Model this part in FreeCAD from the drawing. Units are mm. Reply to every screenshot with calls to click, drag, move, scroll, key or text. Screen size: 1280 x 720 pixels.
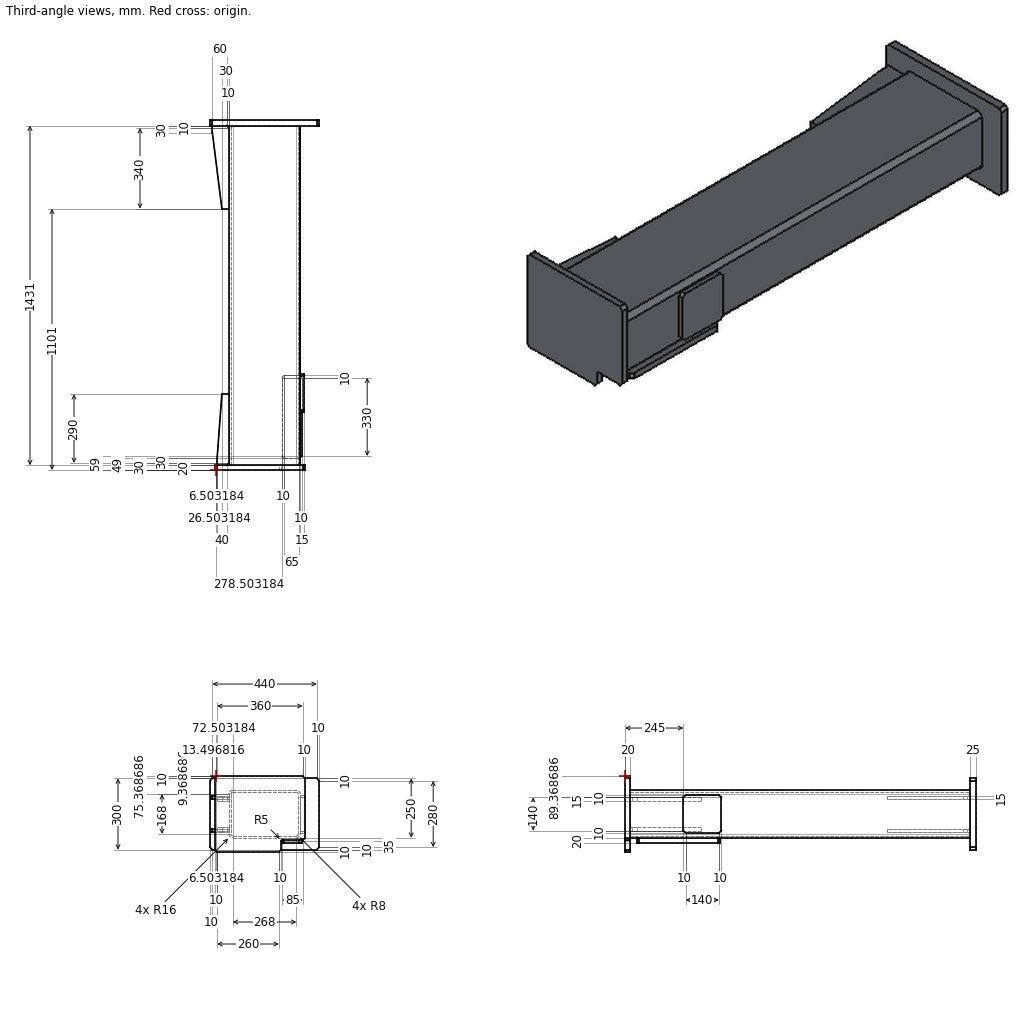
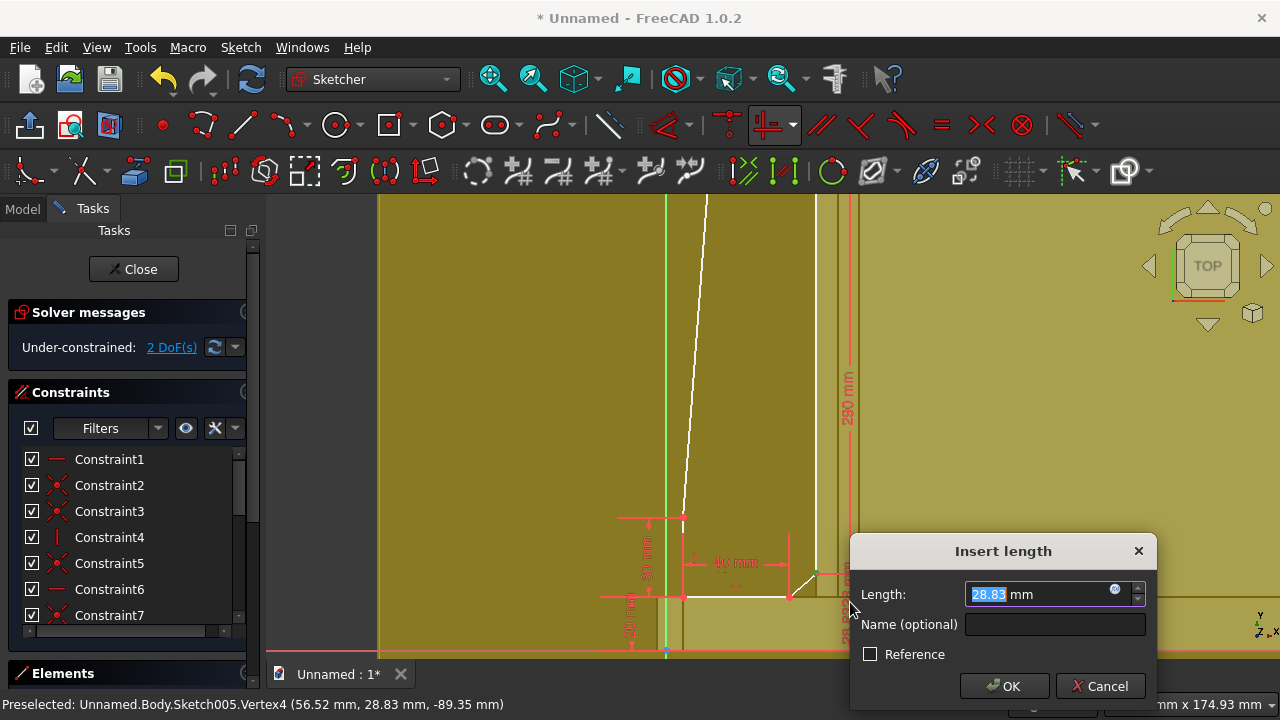
text(30)
key(Return)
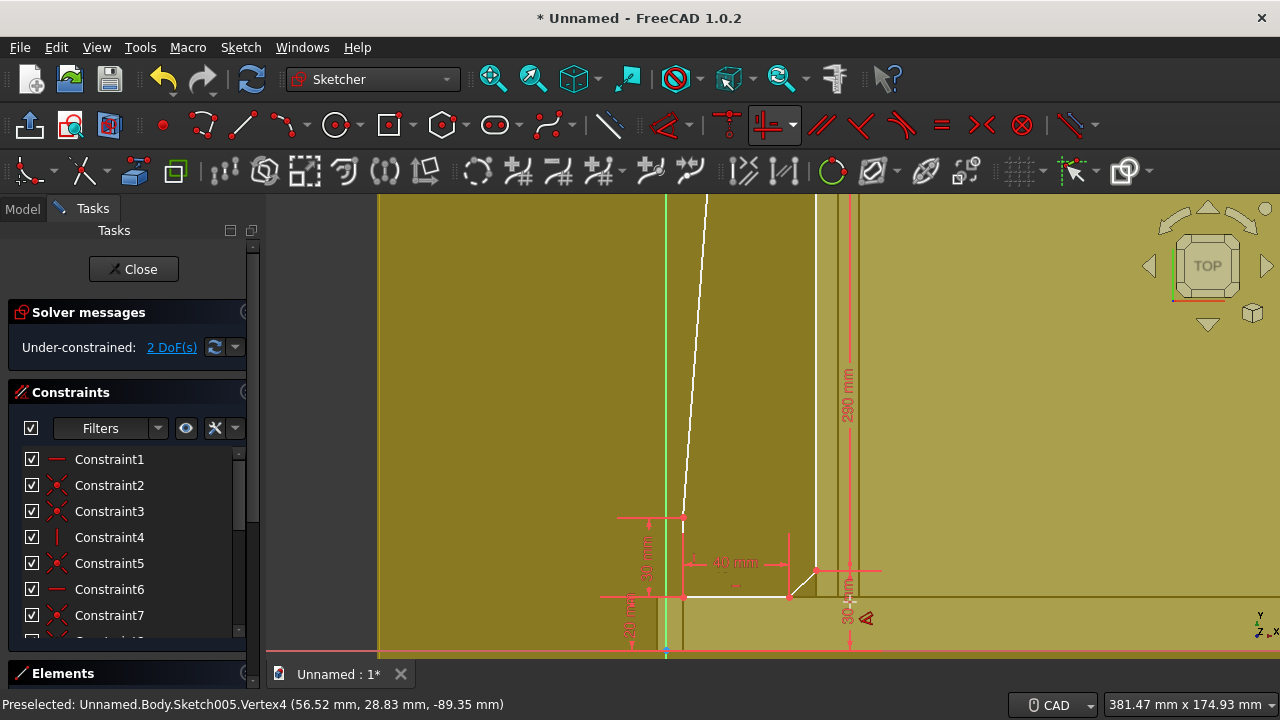
scroll(797, 589, up, 3)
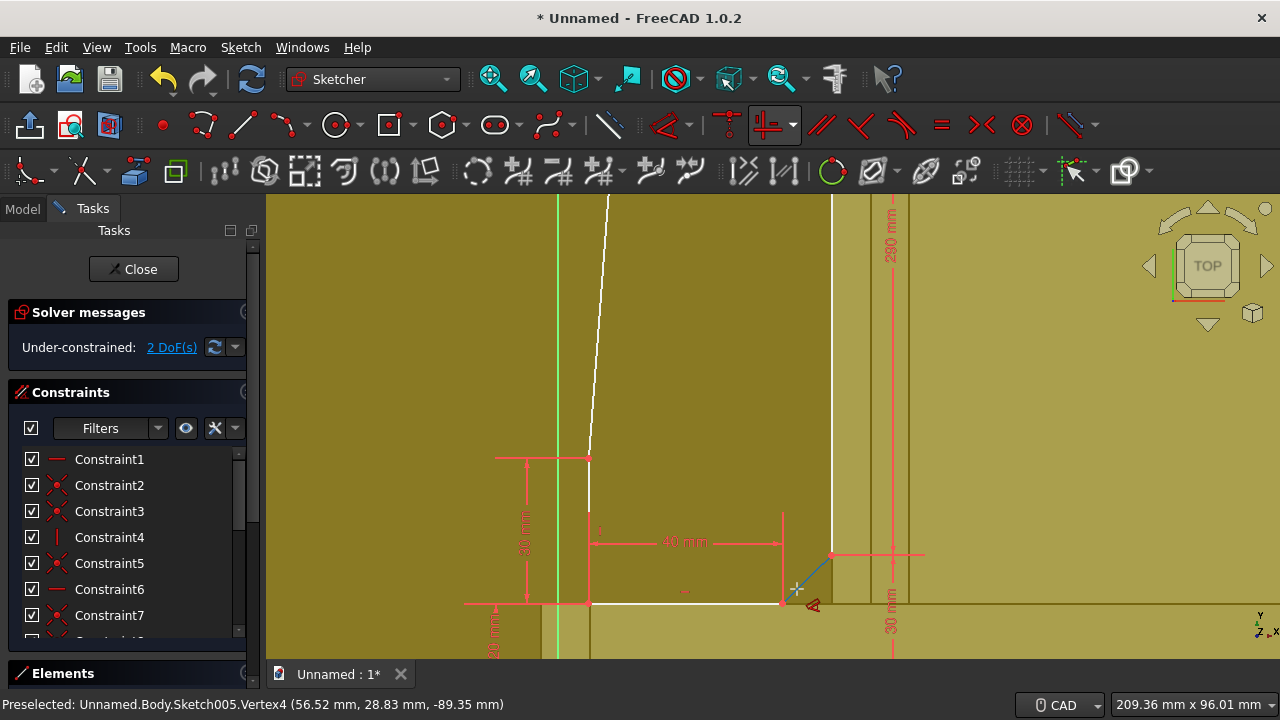
click(797, 589)
click(807, 521)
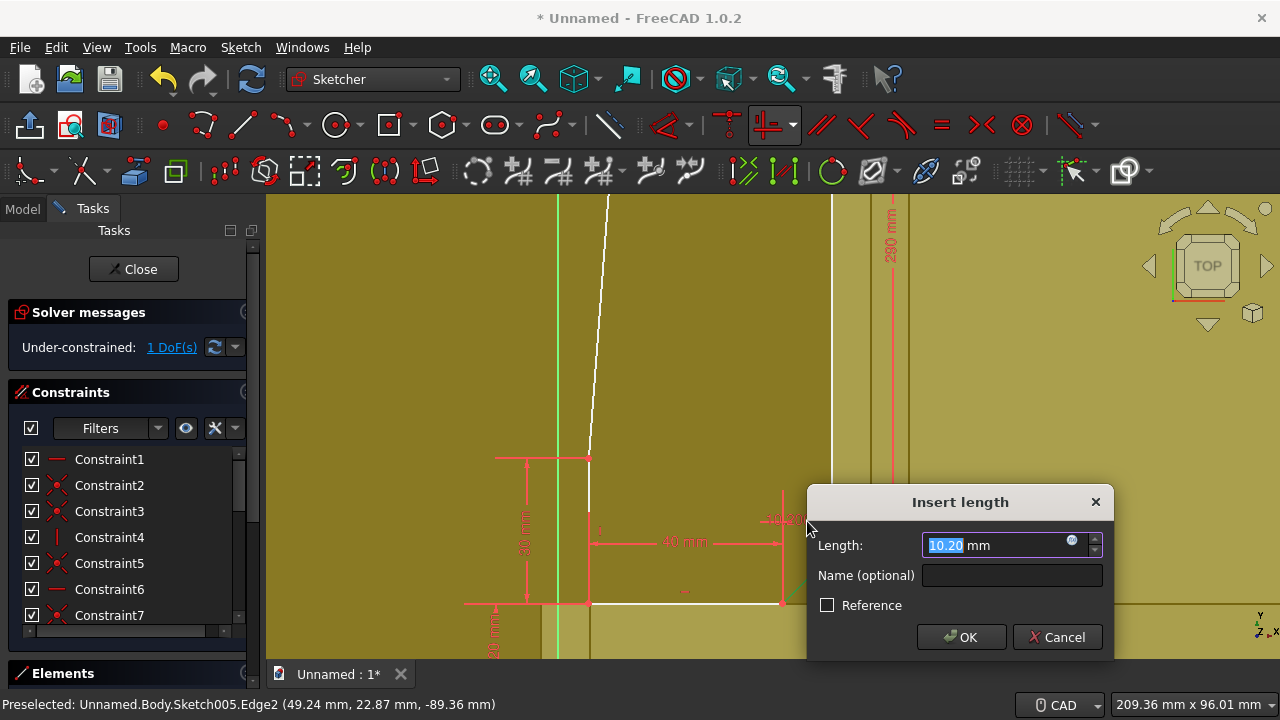
text(10)
key(Return)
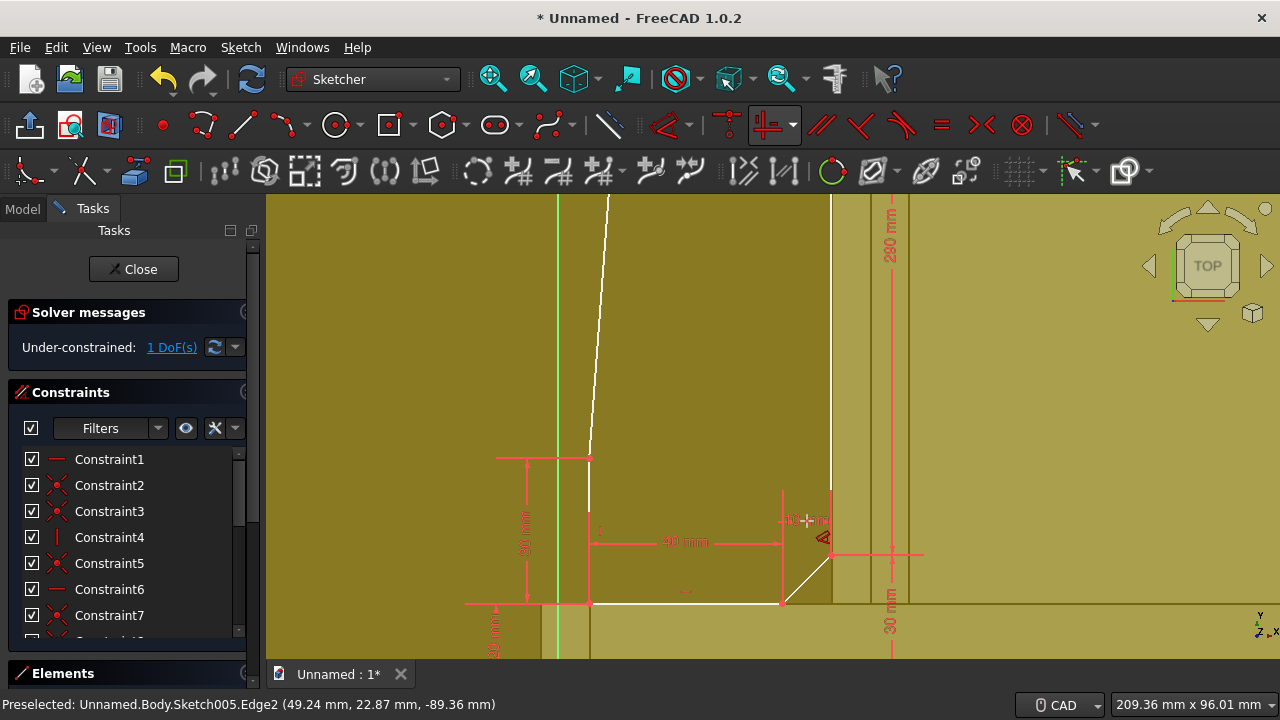
scroll(589, 604, up, 2)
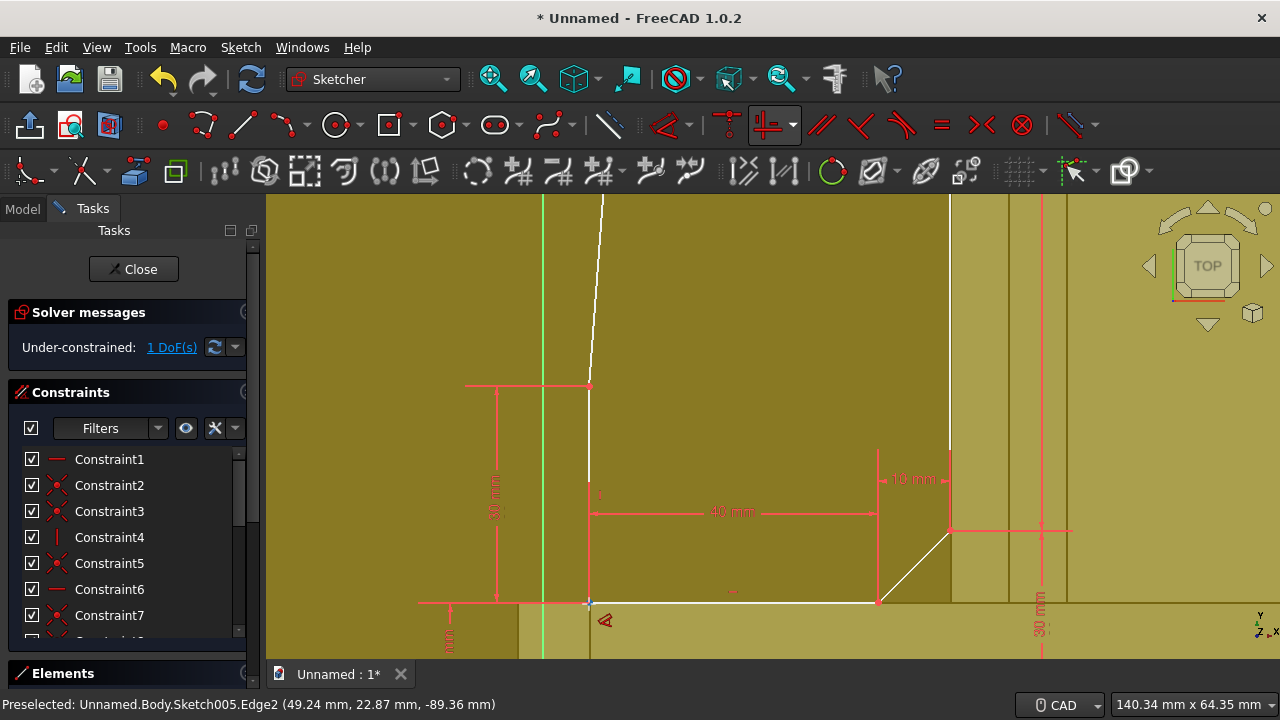
click(589, 603)
click(566, 569)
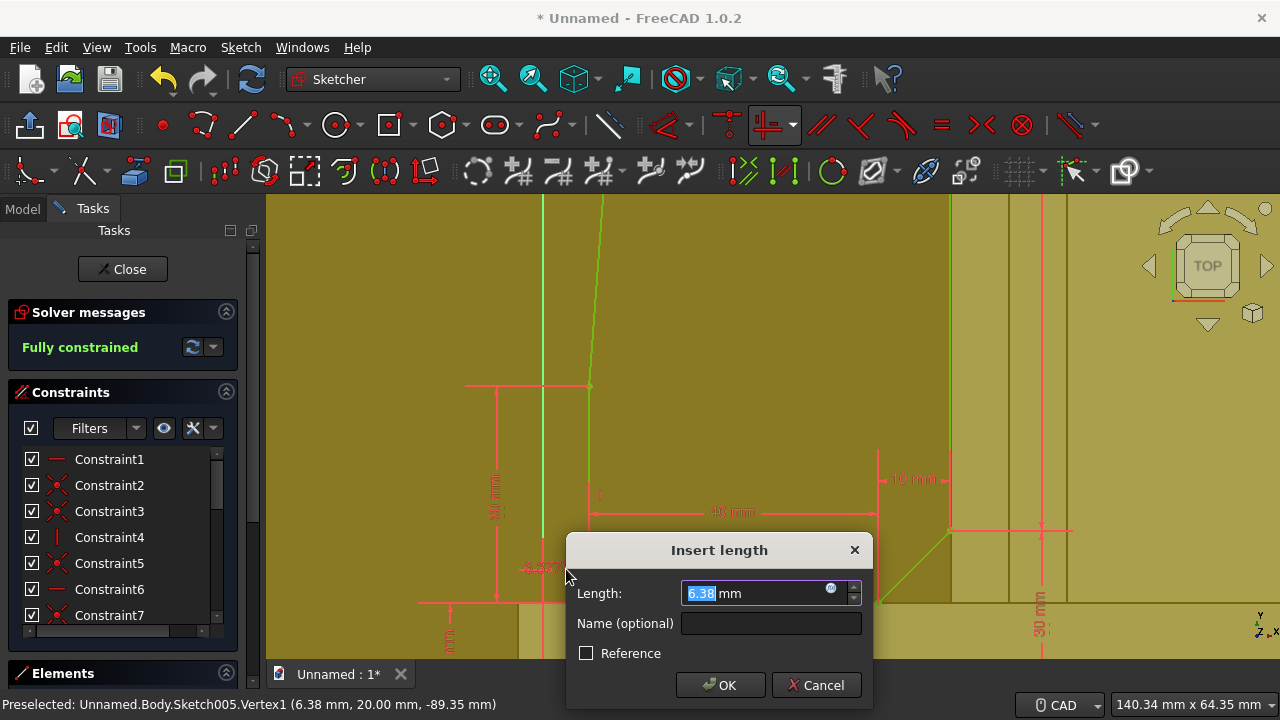
text(6.503184)
key(Return)
key(Escape)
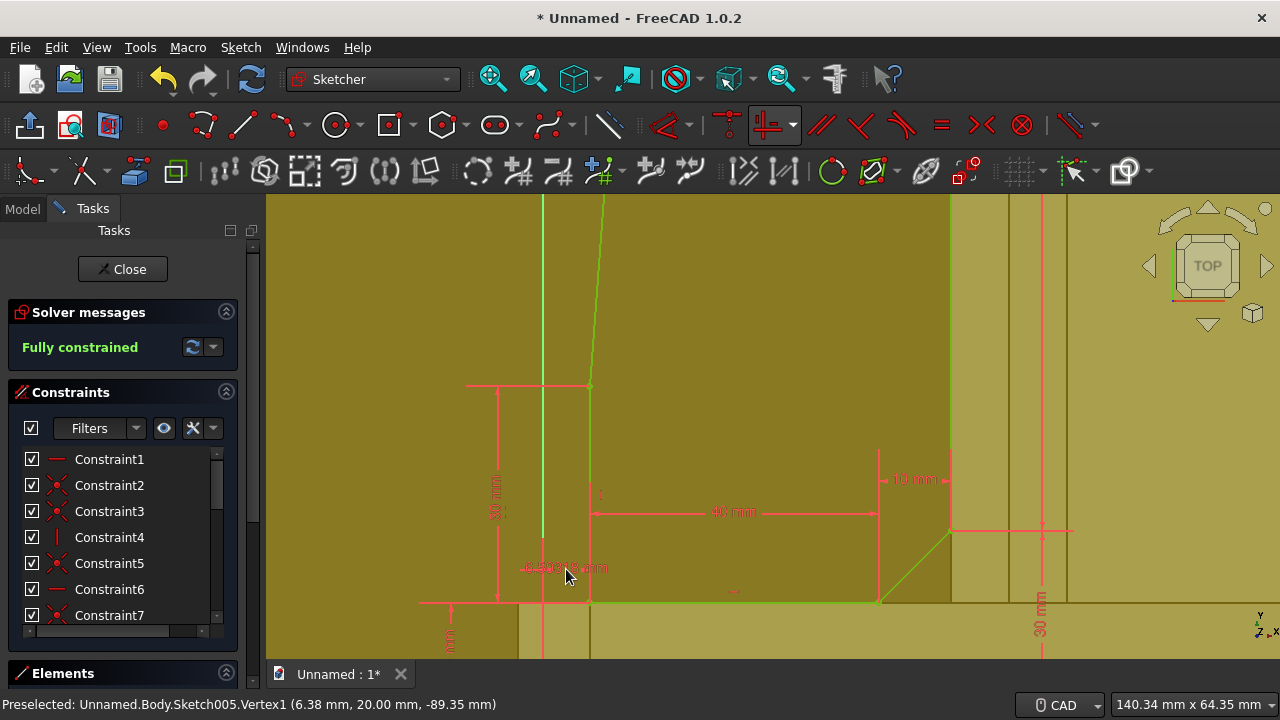
click(123, 269)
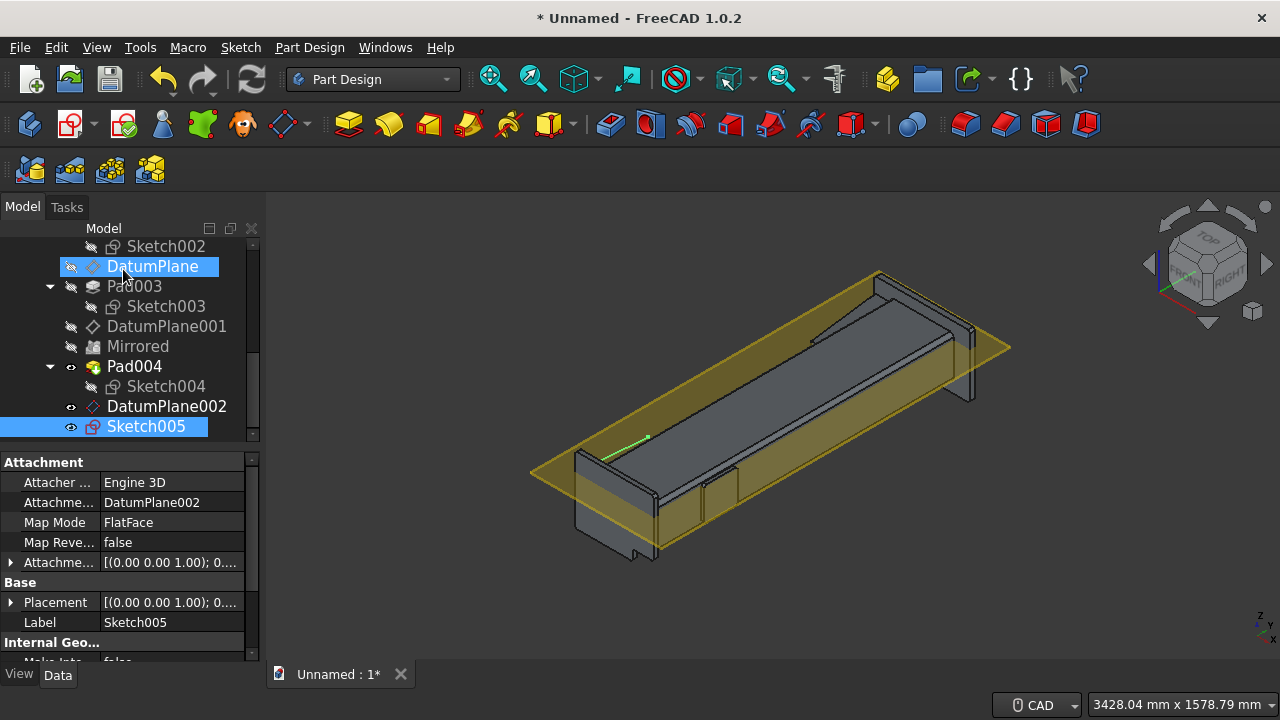
click(350, 124)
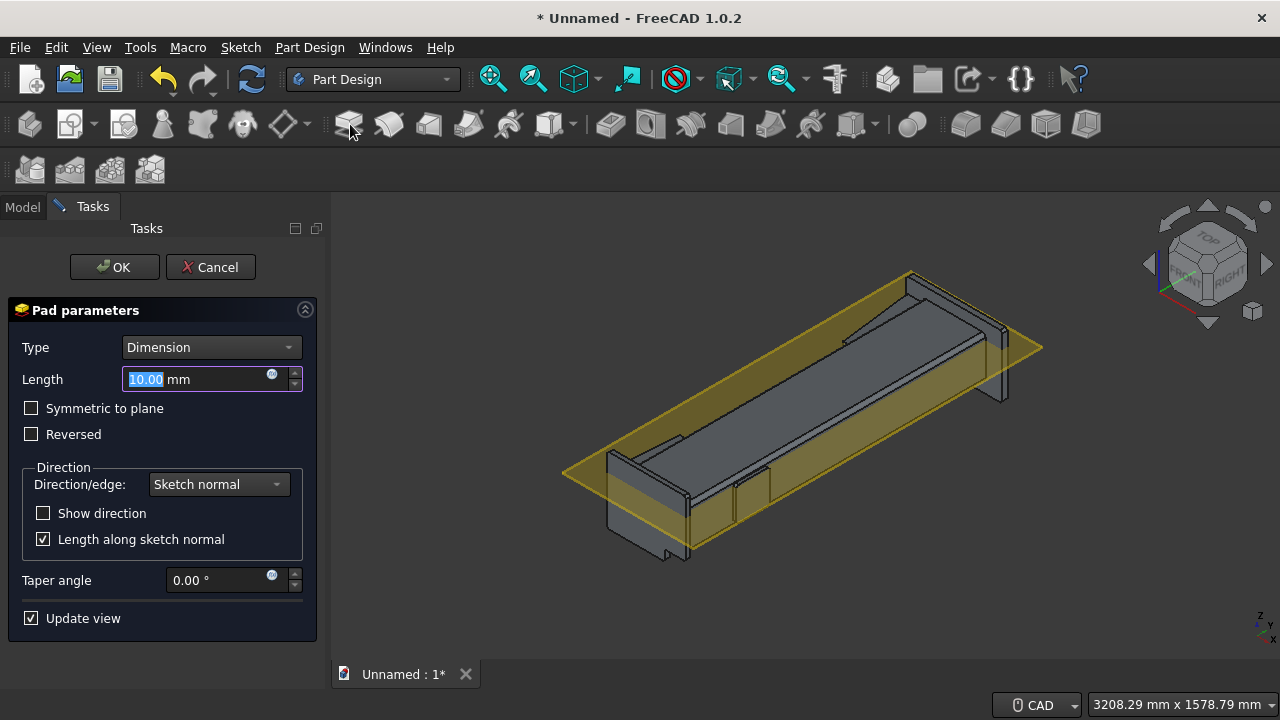
text(15)
key(Tab)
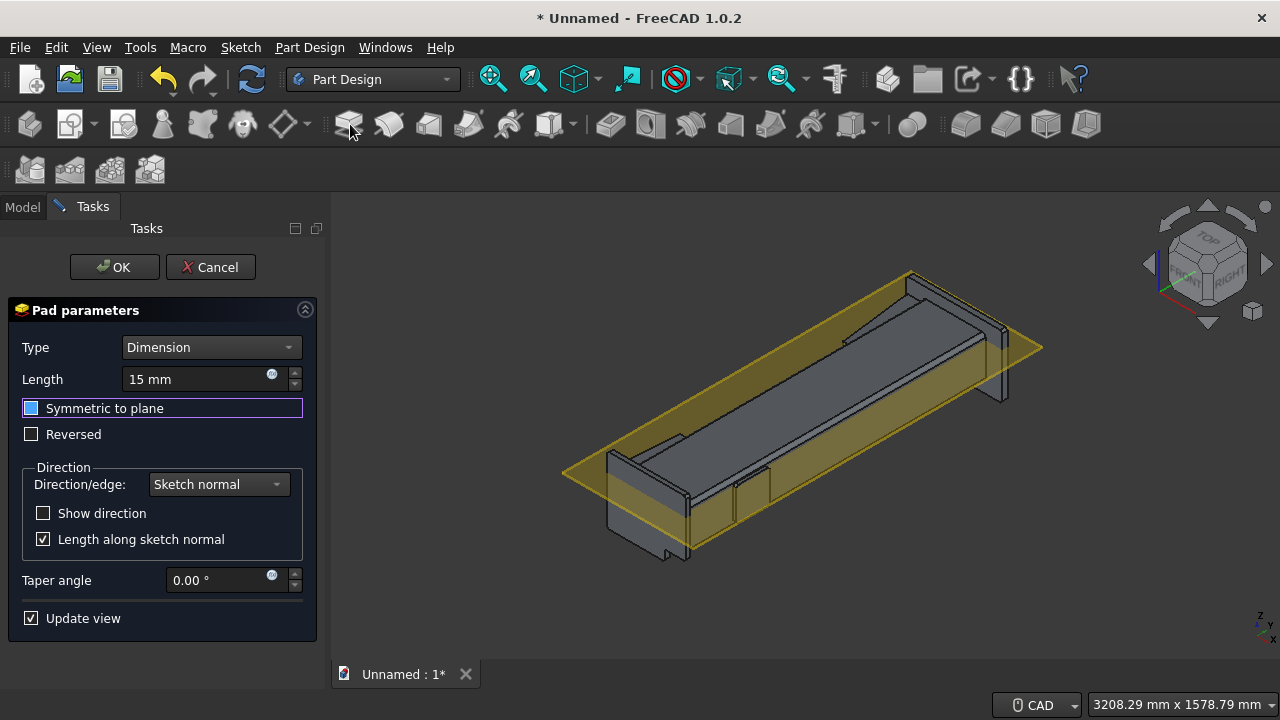
click(30, 434)